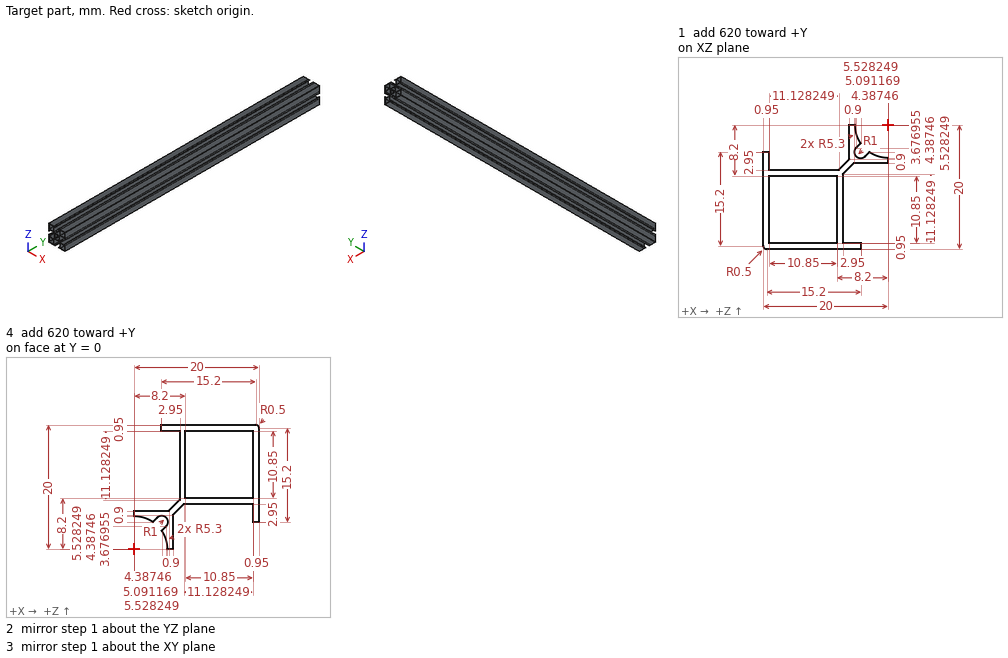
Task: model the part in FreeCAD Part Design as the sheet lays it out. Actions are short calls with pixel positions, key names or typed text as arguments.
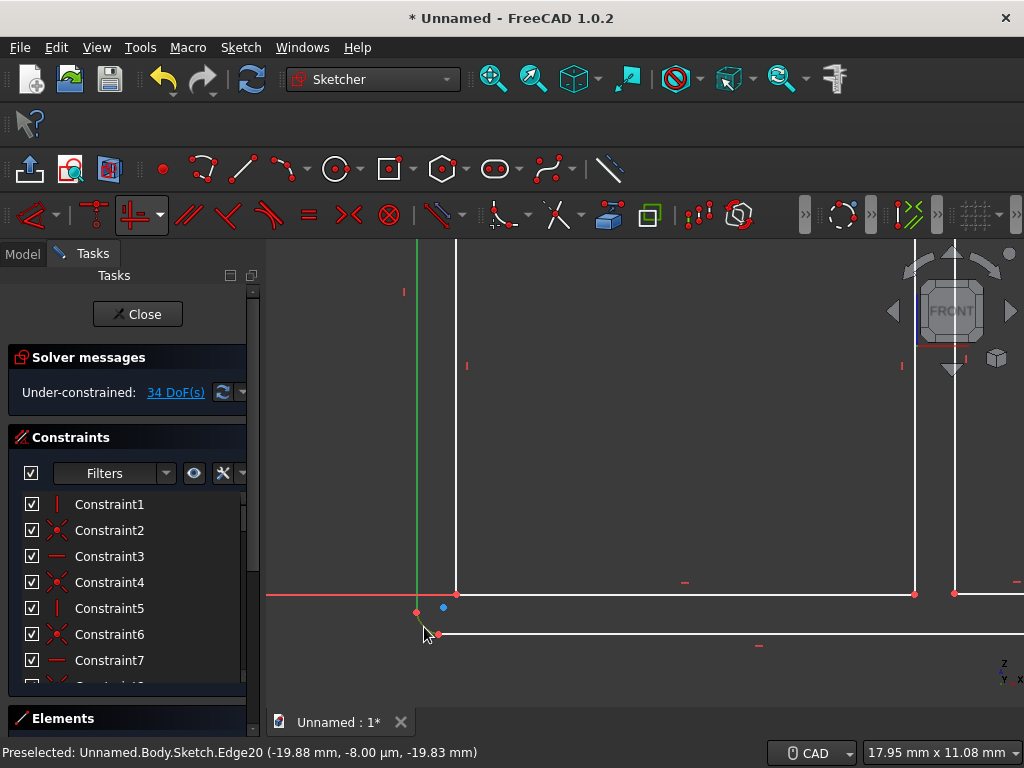
click(270, 216)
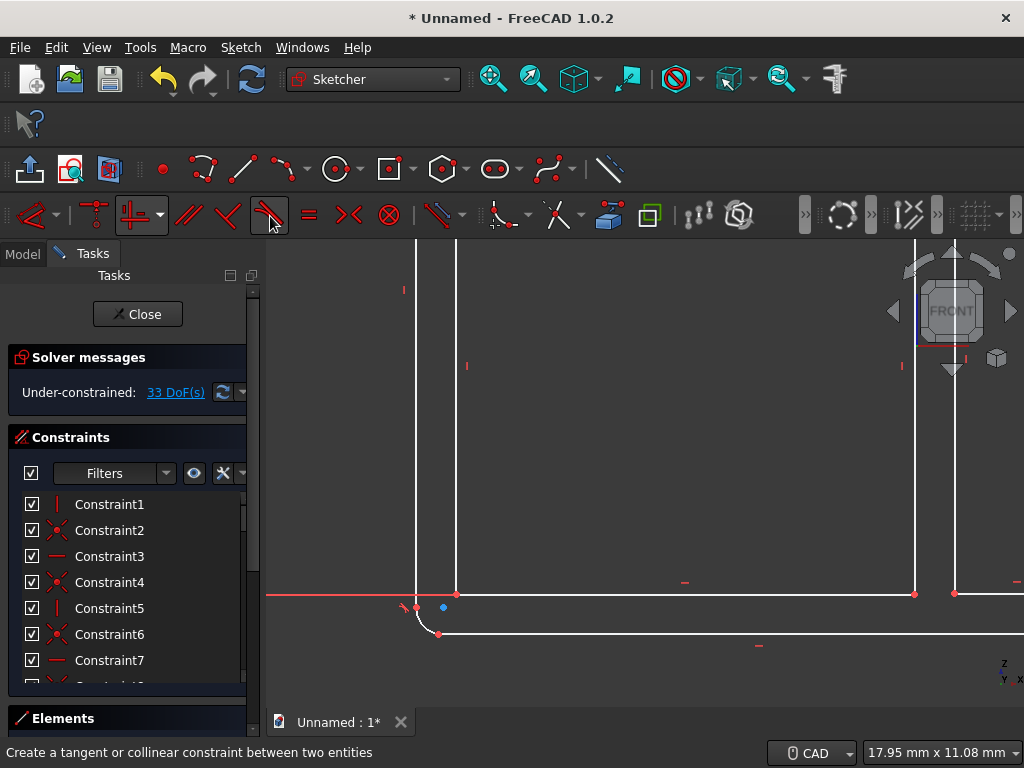
scroll(424, 627, down, 5)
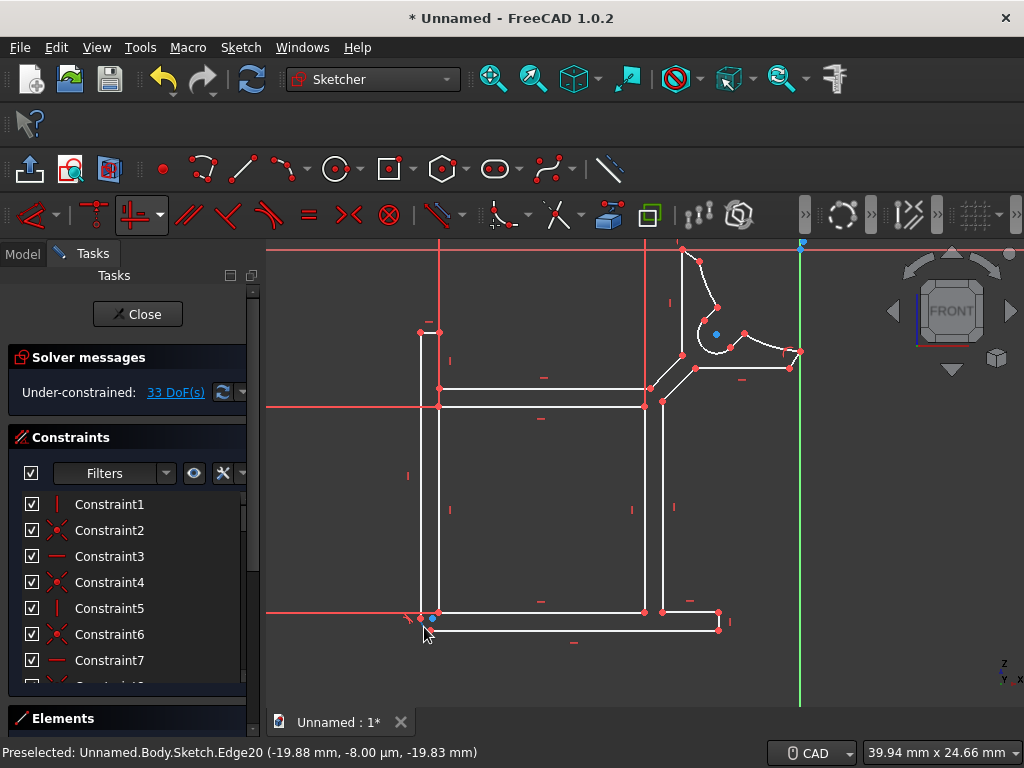
scroll(661, 369, up, 6)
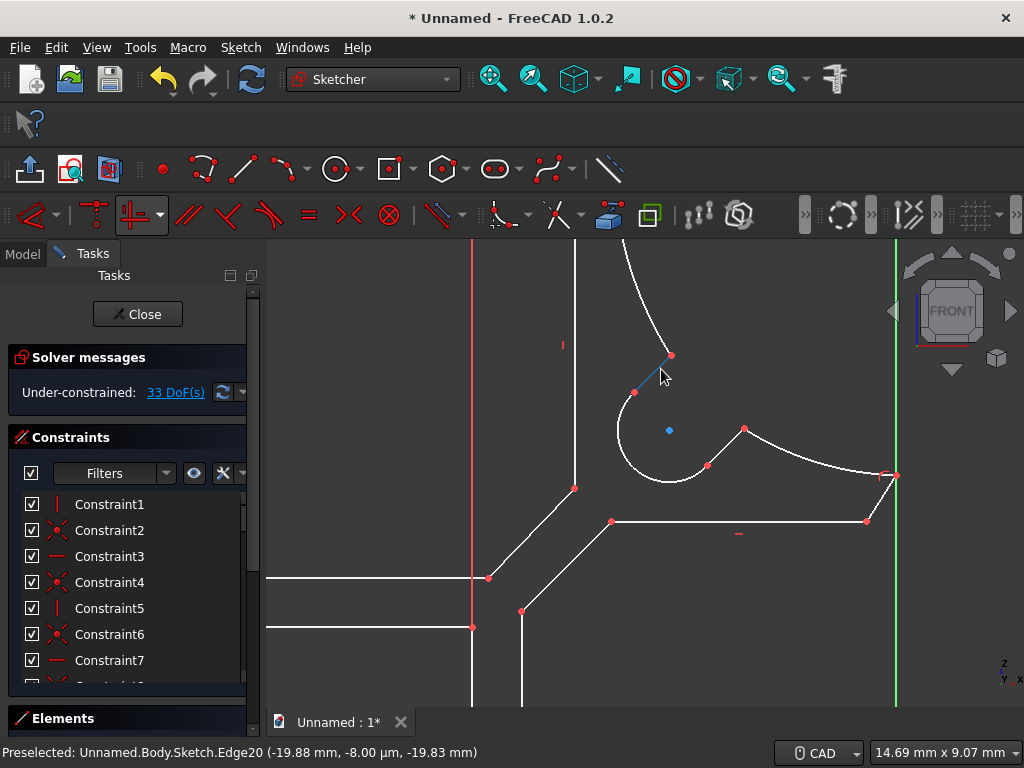
click(660, 367)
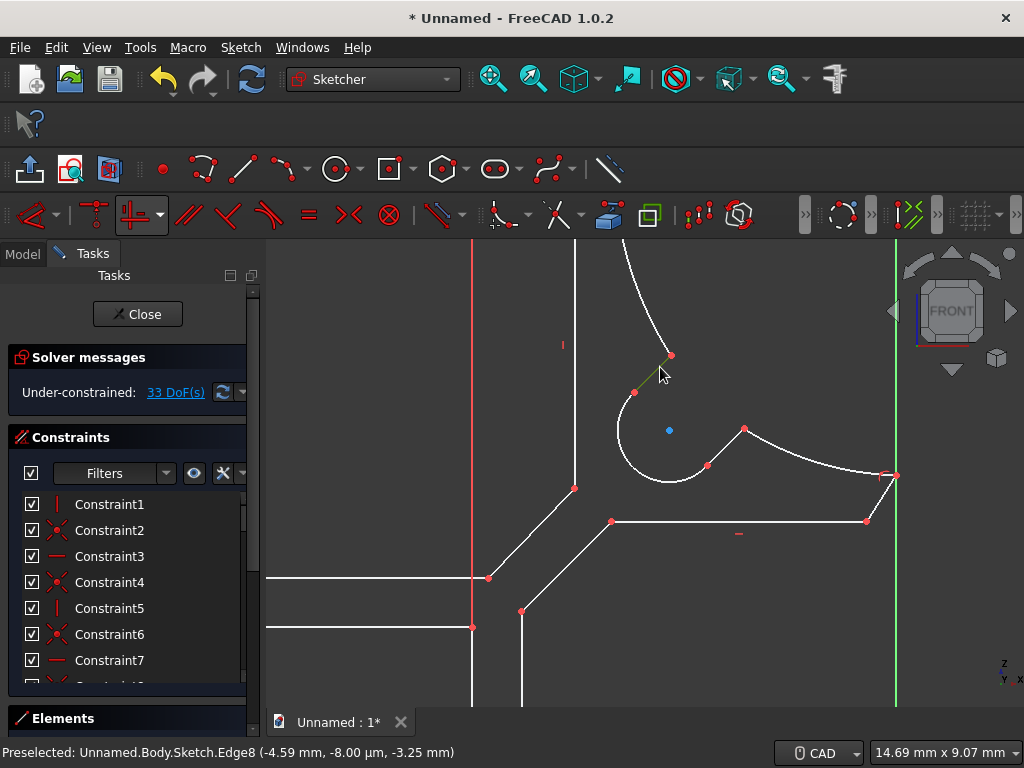
click(618, 438)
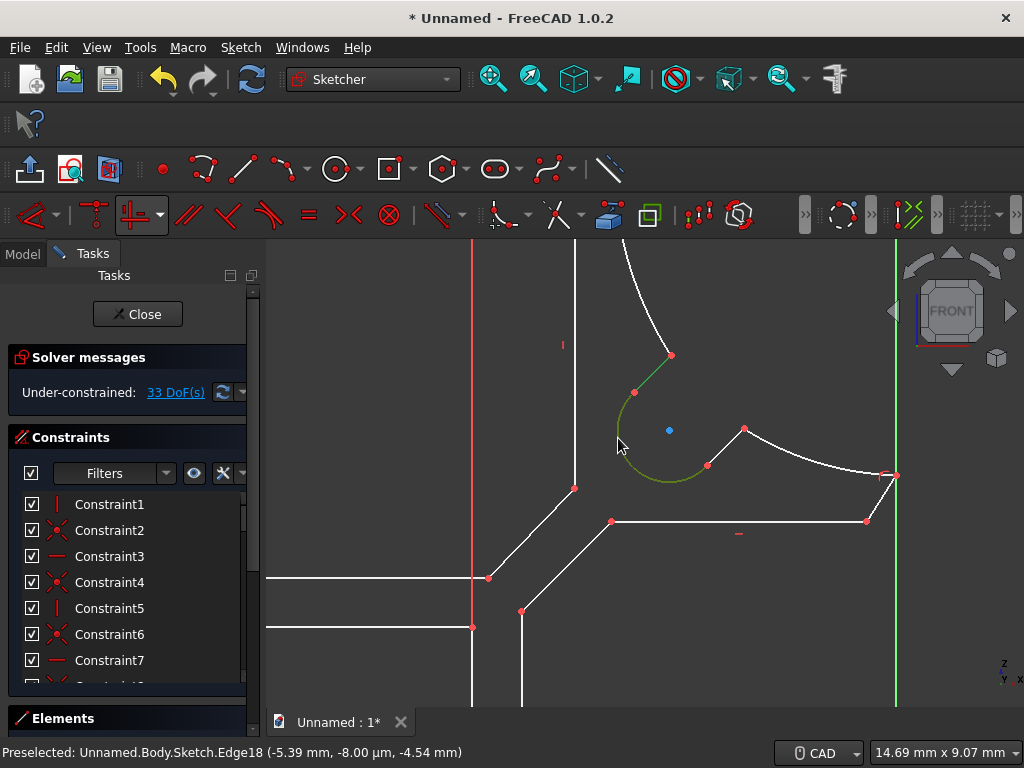
click(270, 216)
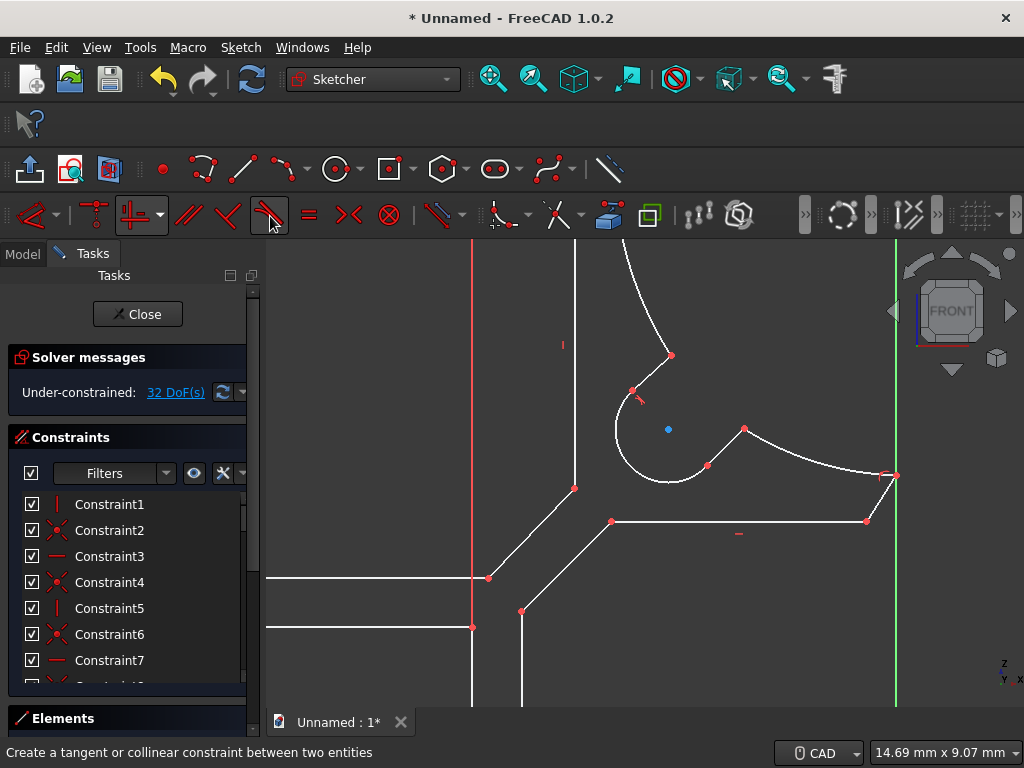
click(718, 454)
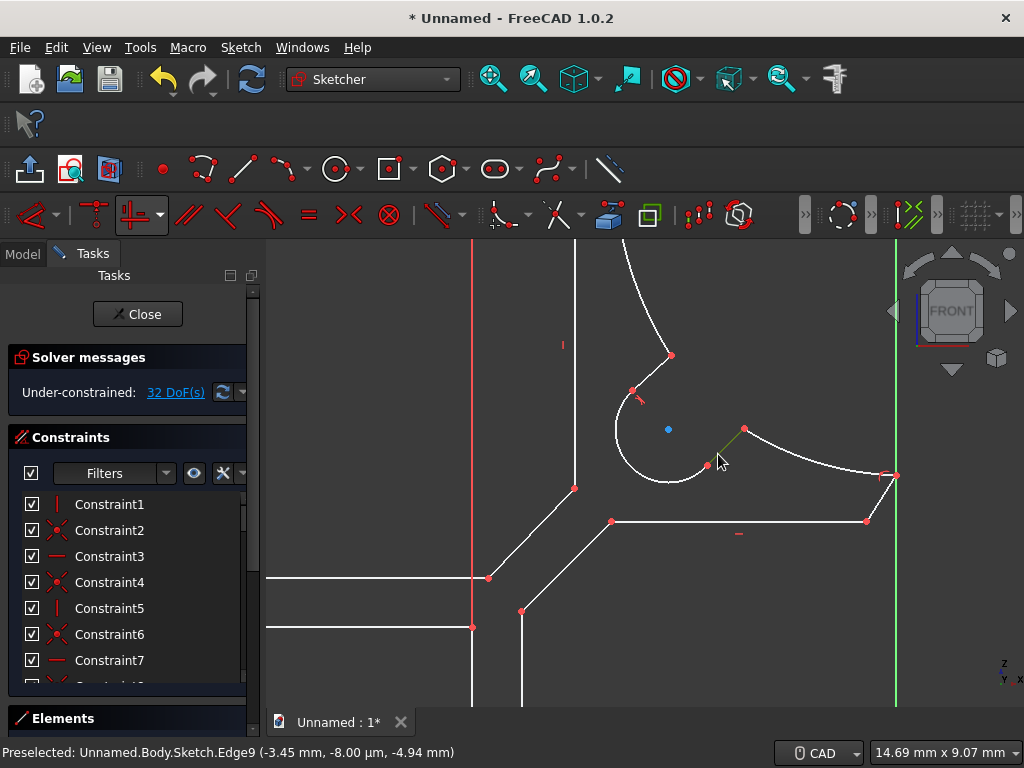
click(616, 437)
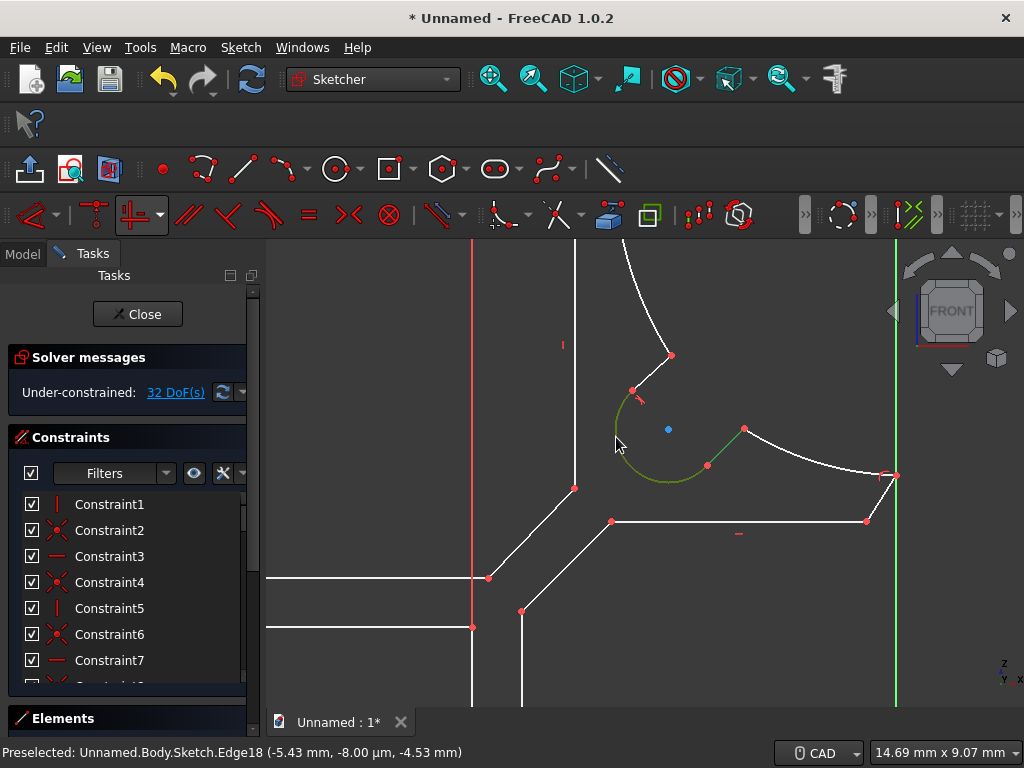
click(270, 216)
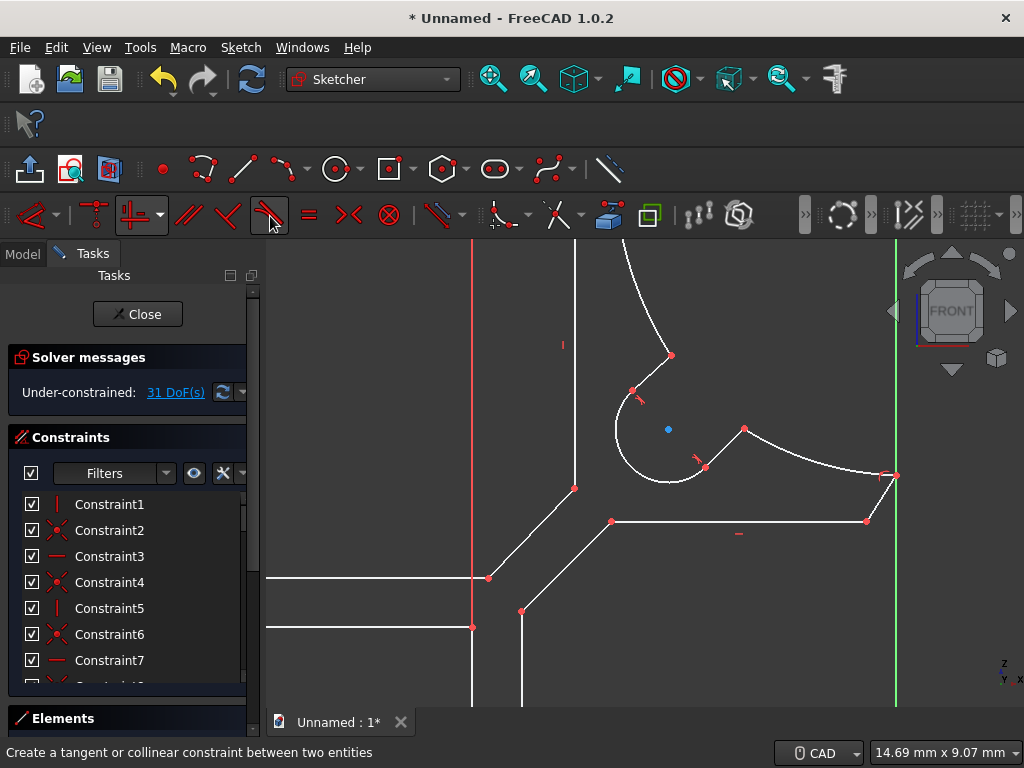
scroll(661, 368, down, 6)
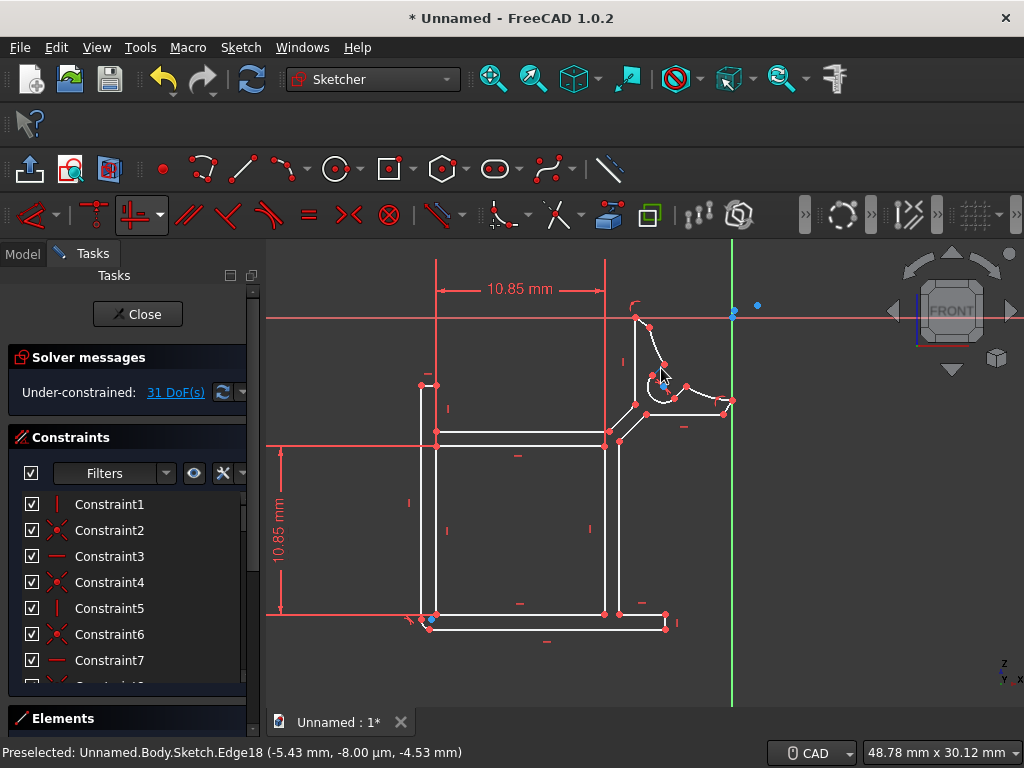
click(595, 630)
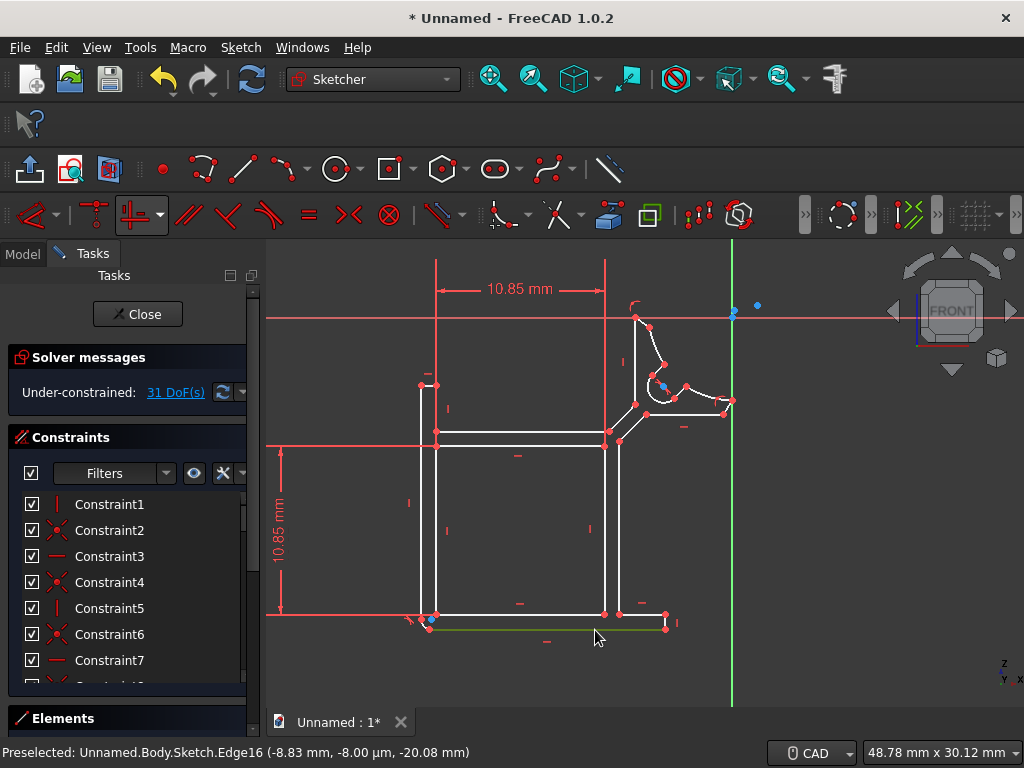
scroll(424, 626, up, 4)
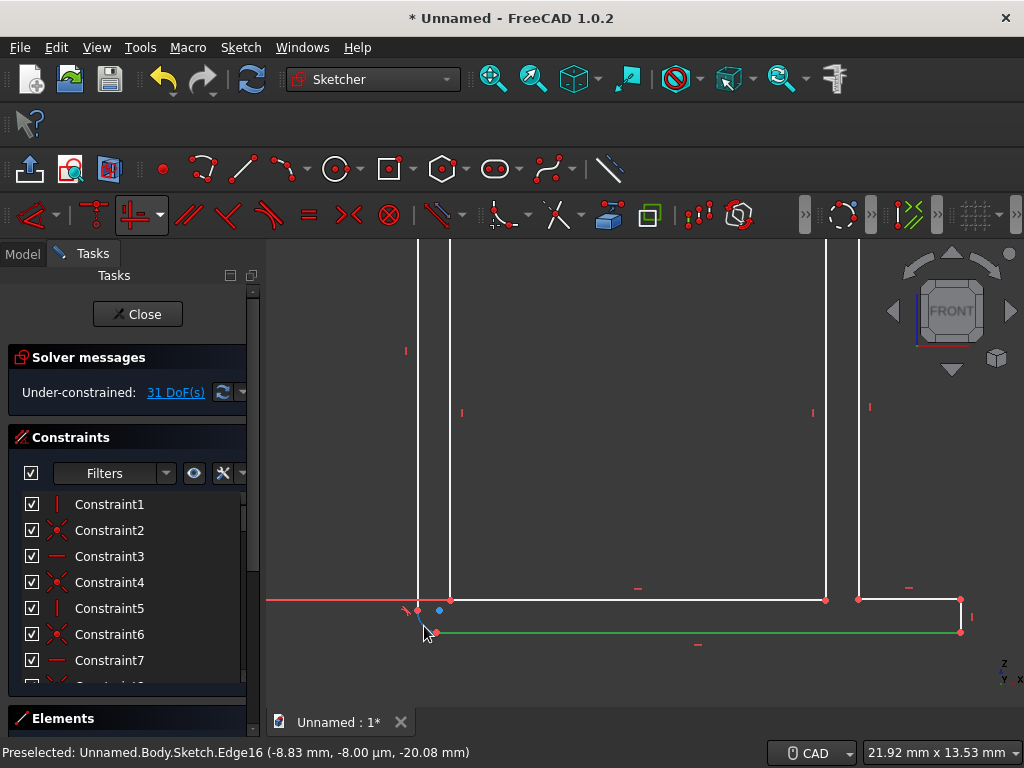
click(423, 625)